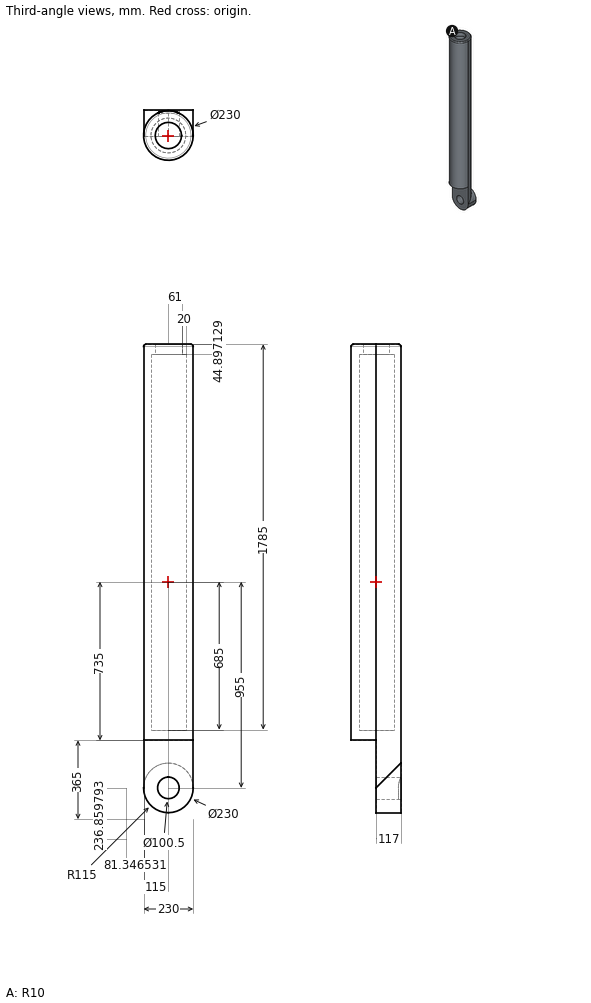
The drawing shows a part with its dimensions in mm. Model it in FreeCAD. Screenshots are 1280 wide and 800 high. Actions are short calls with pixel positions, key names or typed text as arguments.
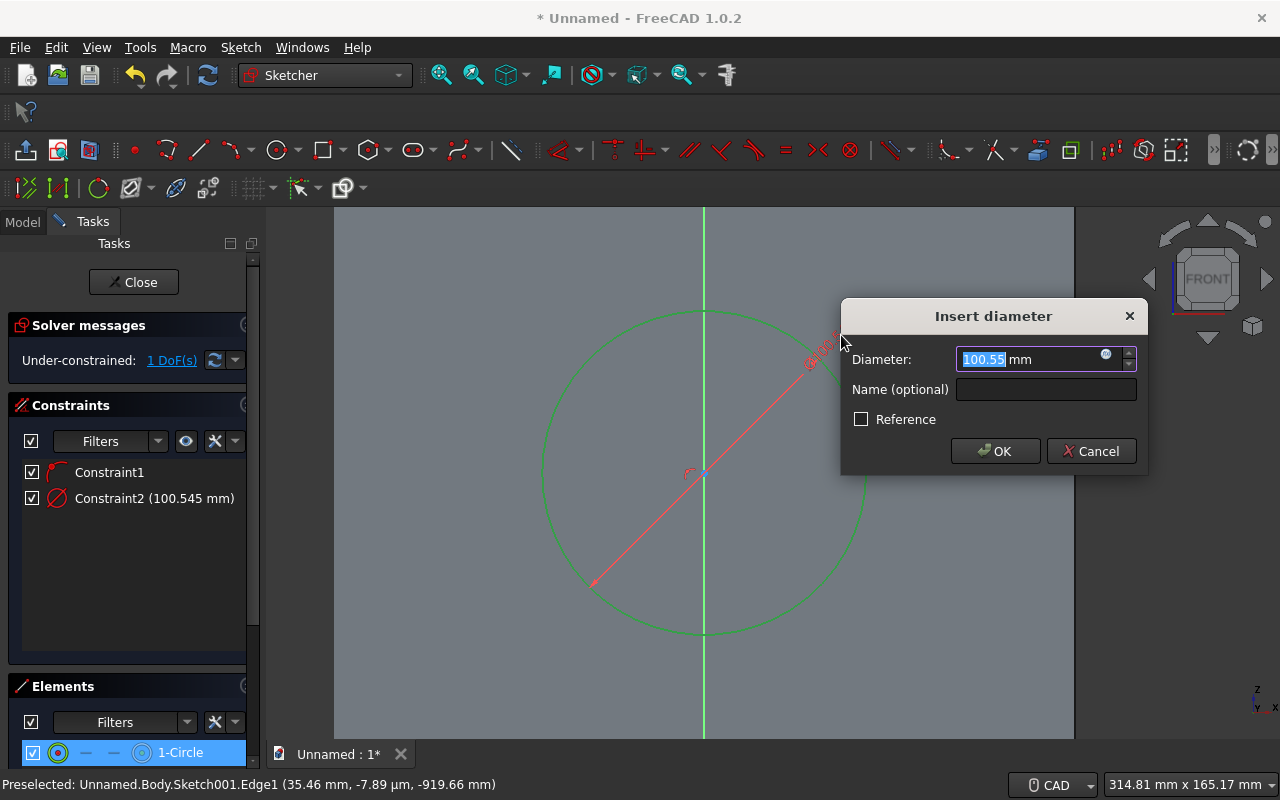
text(100.5)
key(Return)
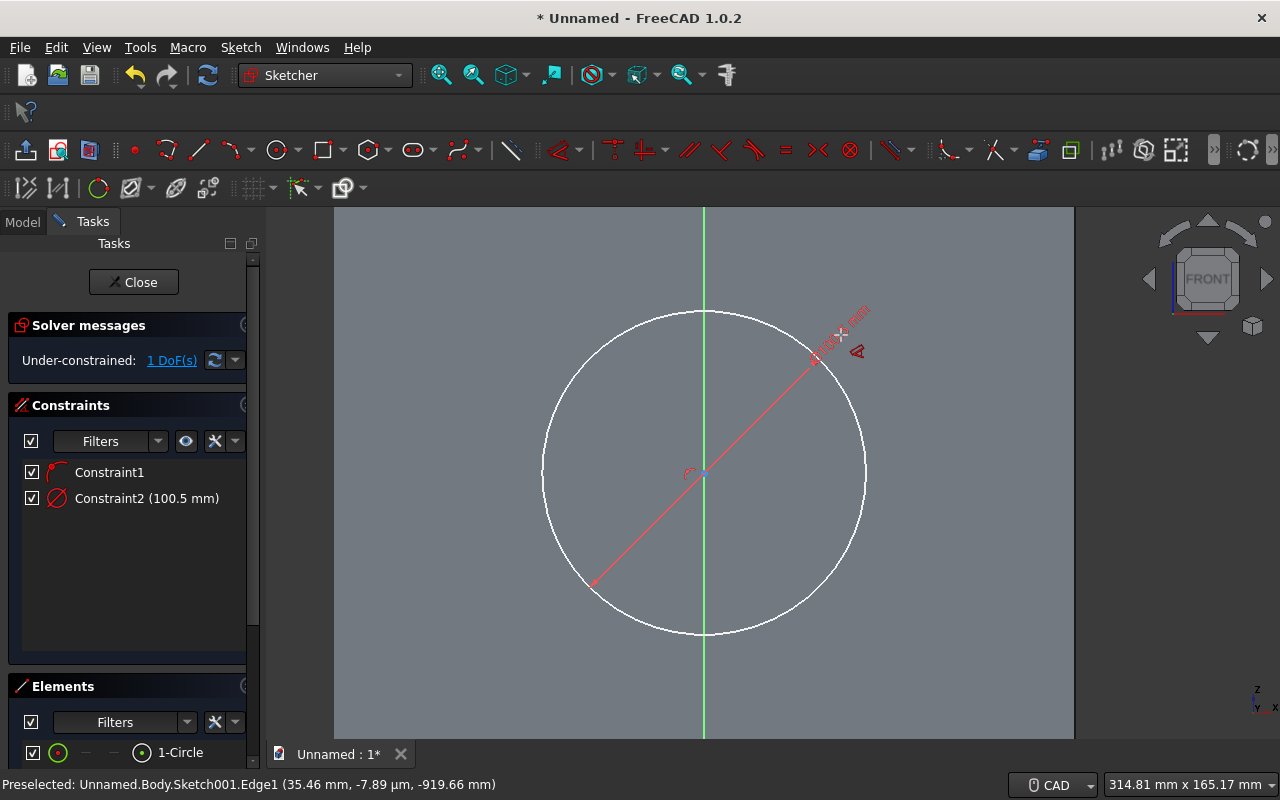
click(704, 473)
click(738, 354)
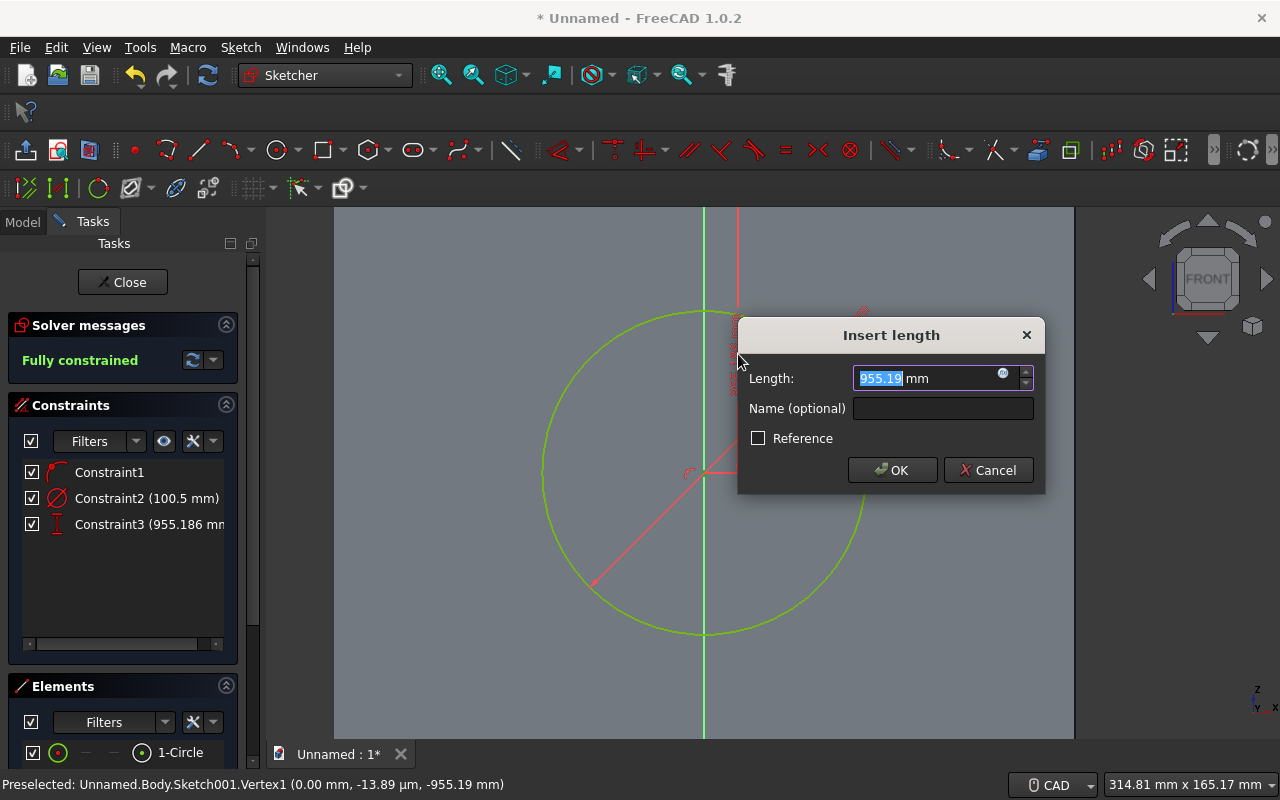
text(955)
key(Return)
key(Escape)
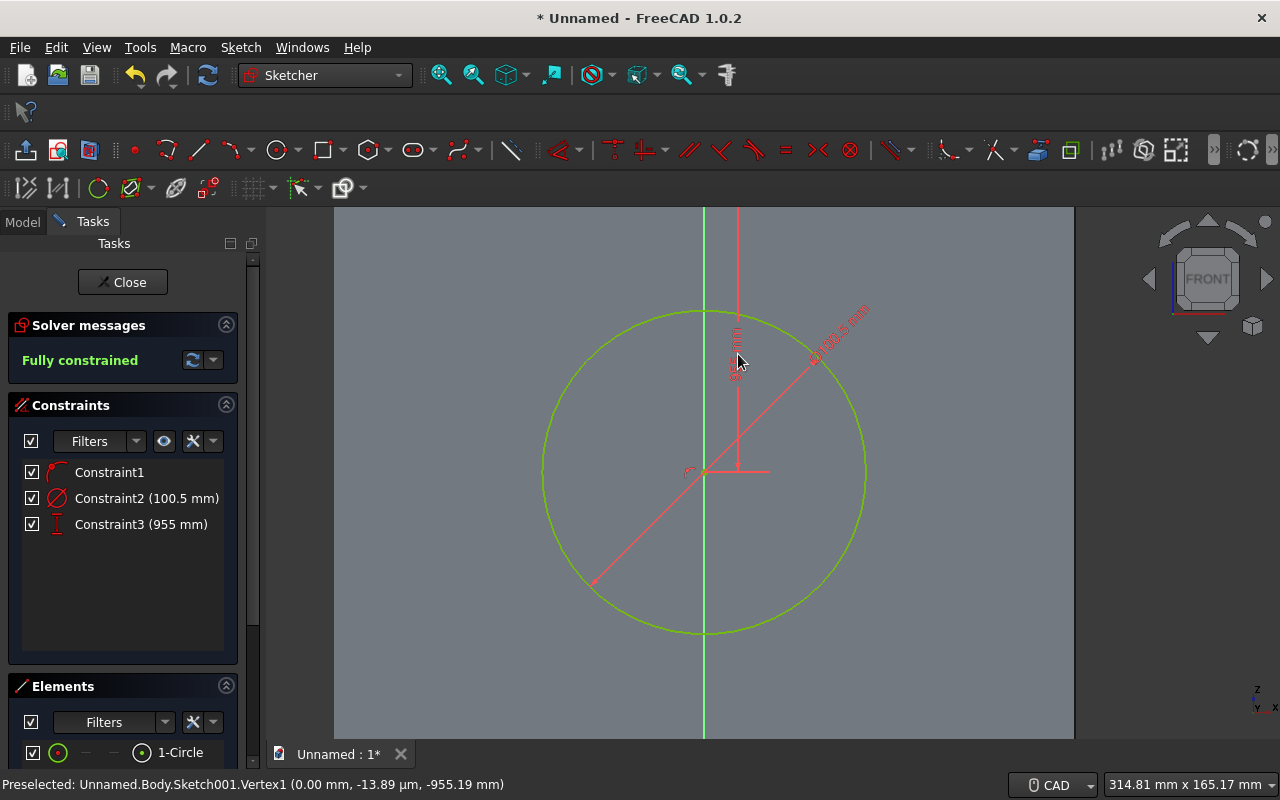
click(123, 282)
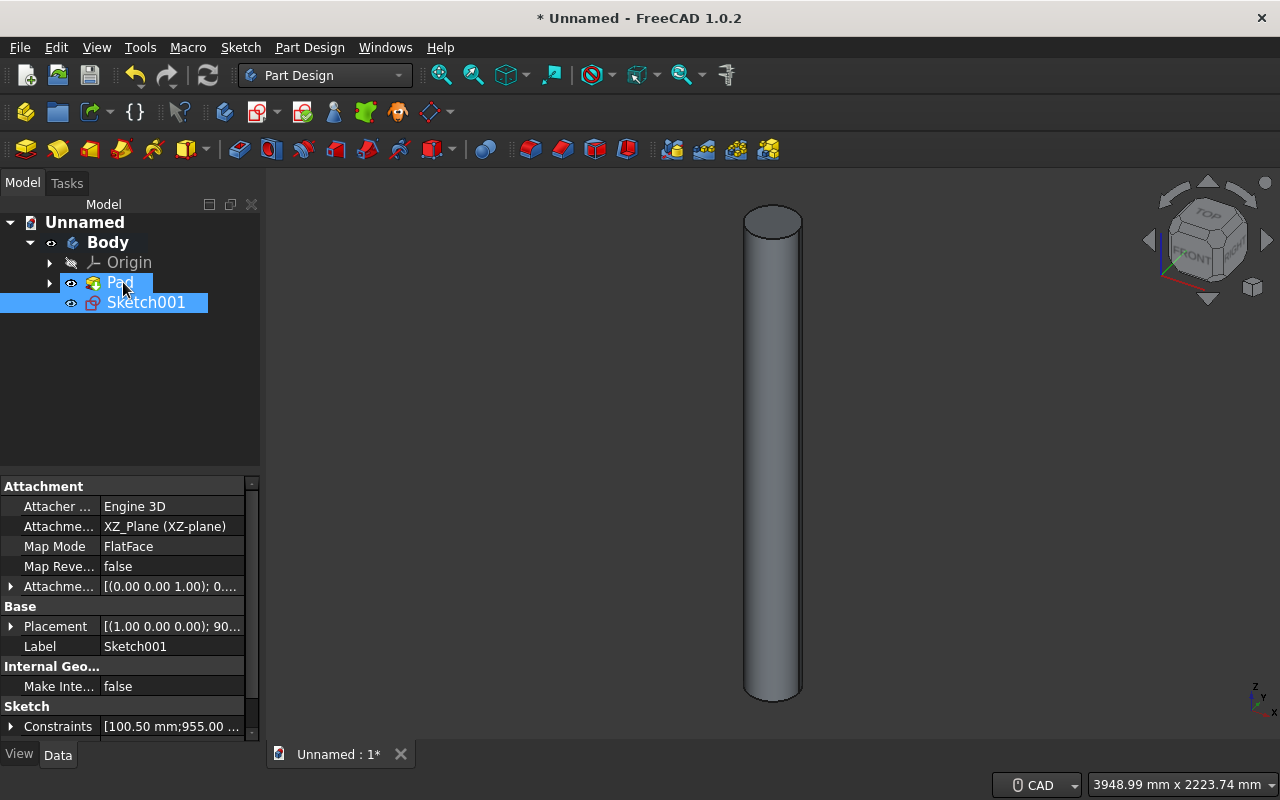
click(240, 150)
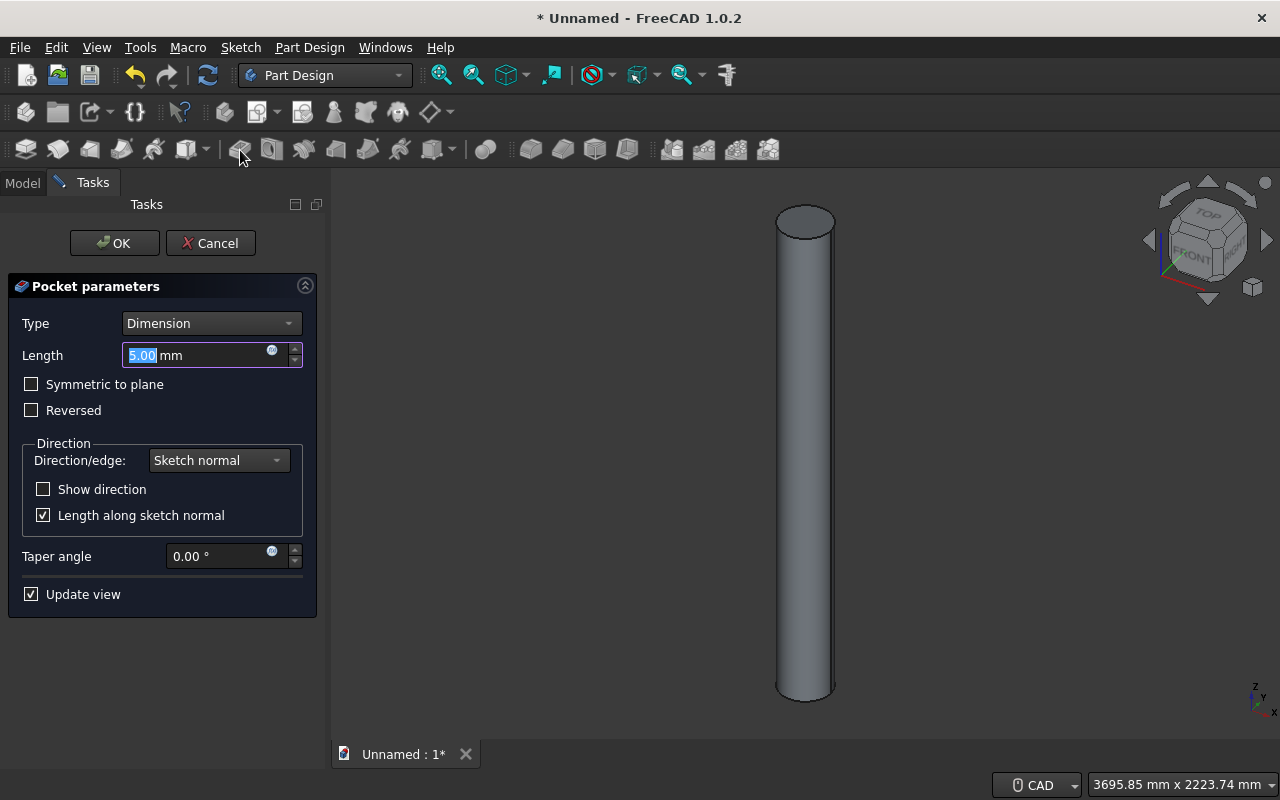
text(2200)
key(Tab)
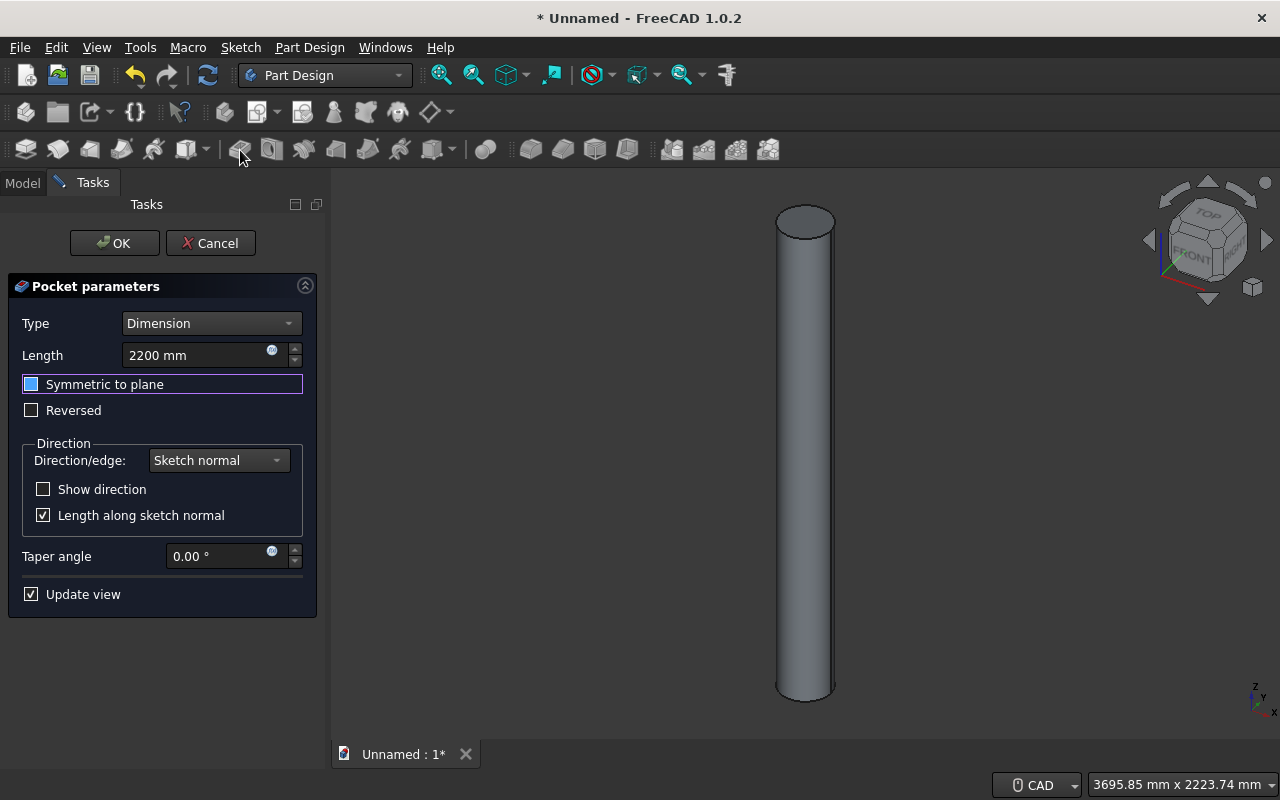
click(30, 384)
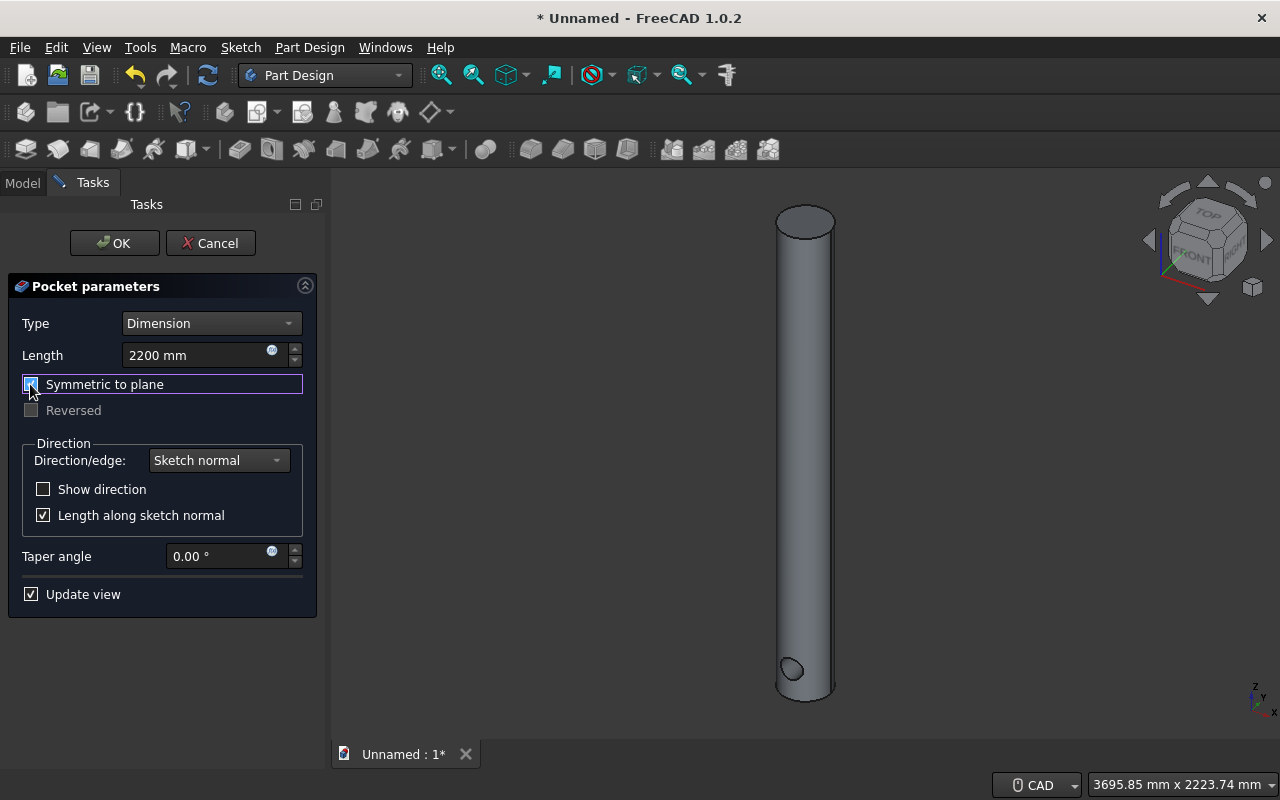
click(115, 243)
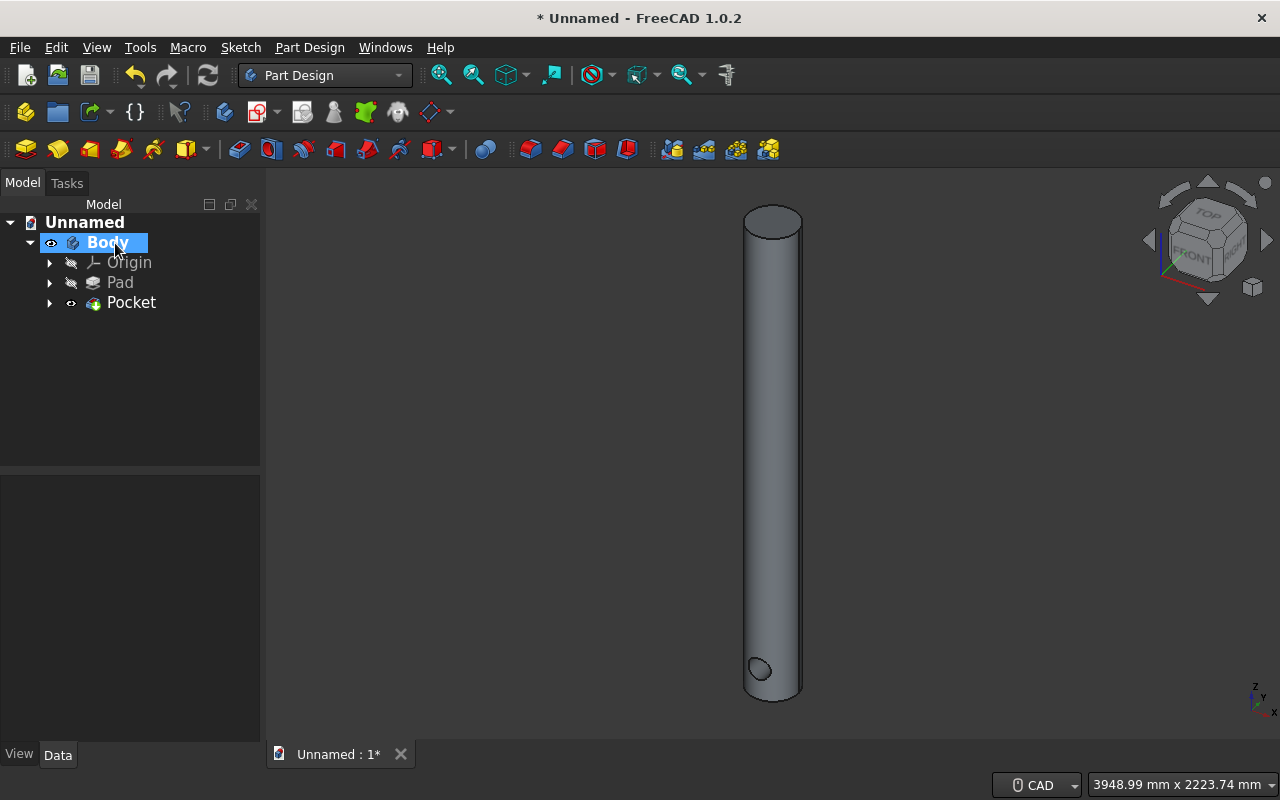
click(258, 112)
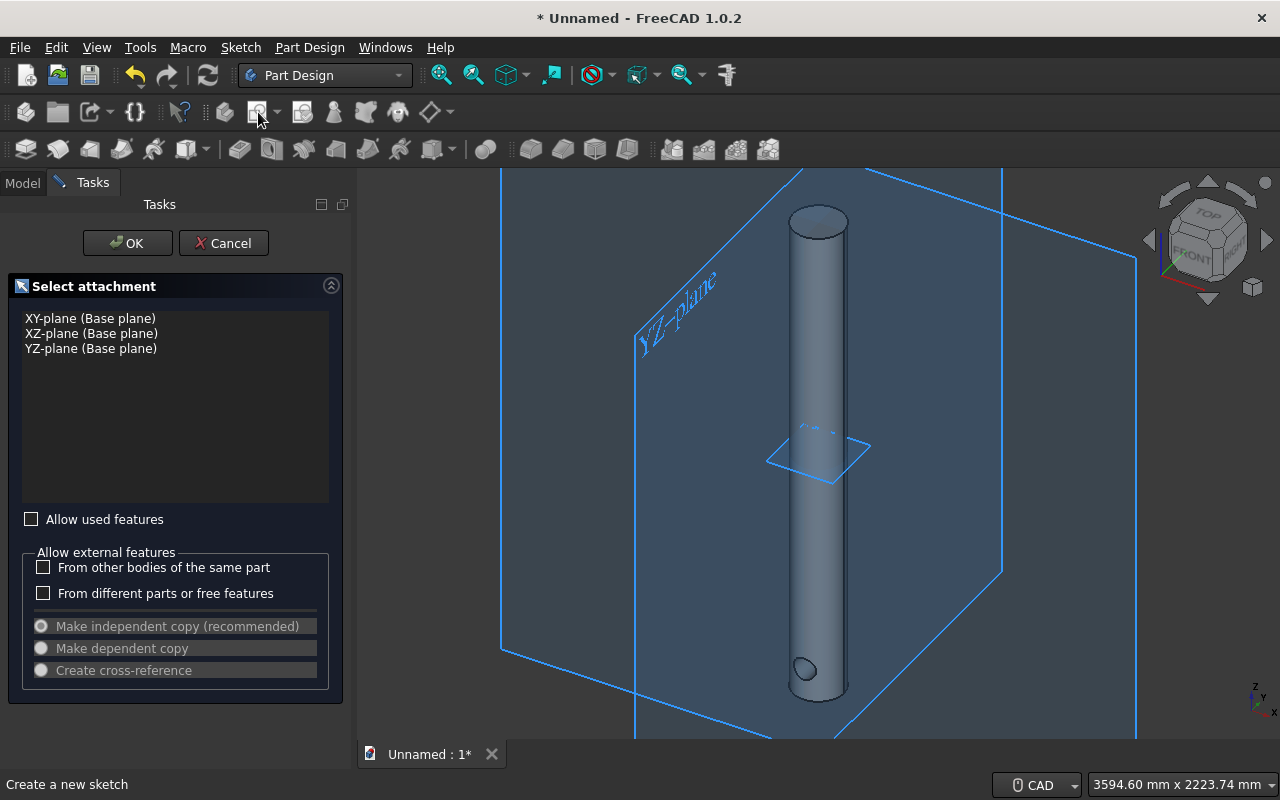
click(82, 334)